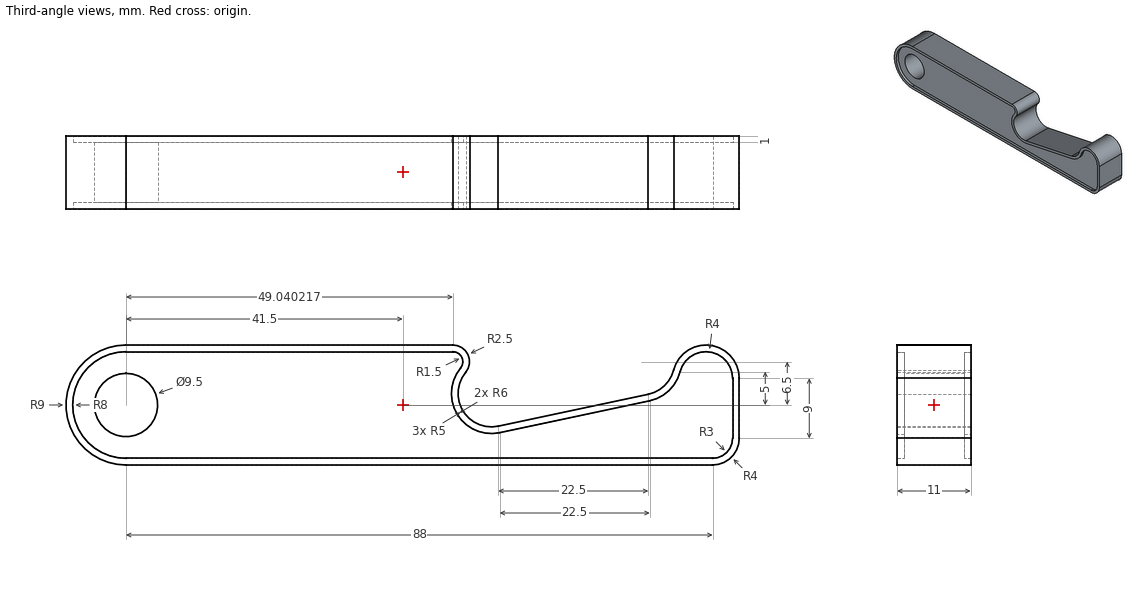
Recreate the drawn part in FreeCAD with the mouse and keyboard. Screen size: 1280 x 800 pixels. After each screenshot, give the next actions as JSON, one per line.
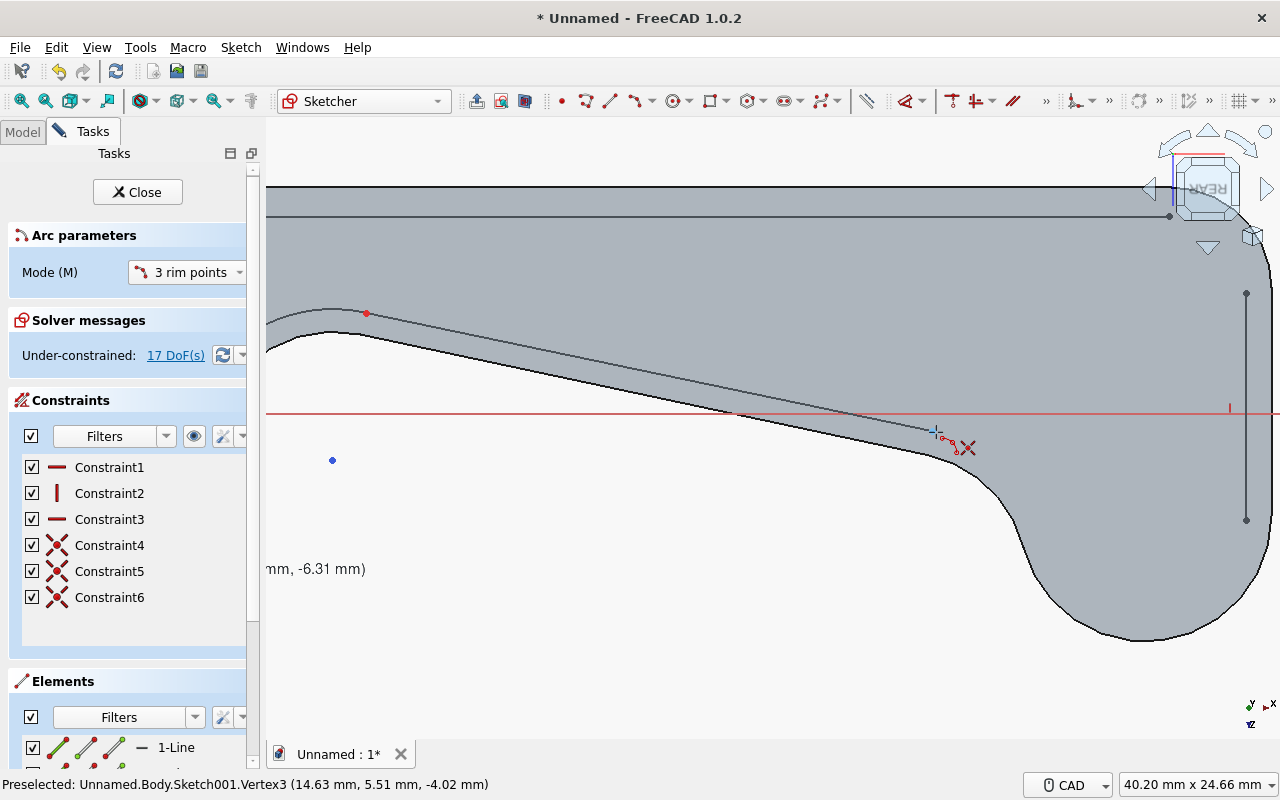
{"action": "left_click", "coordinate": [933, 431]}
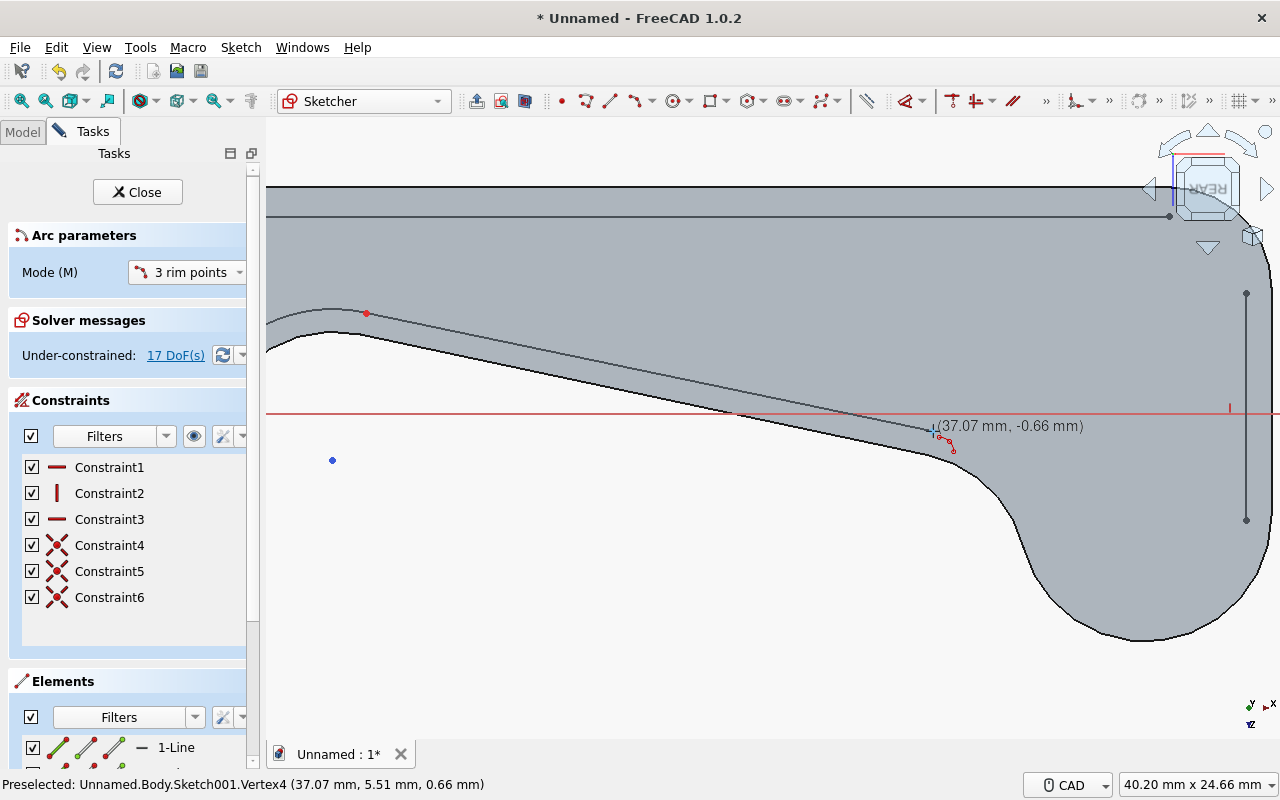
{"action": "scroll", "coordinate": [936, 432], "scroll_direction": "down", "scroll_amount": 7}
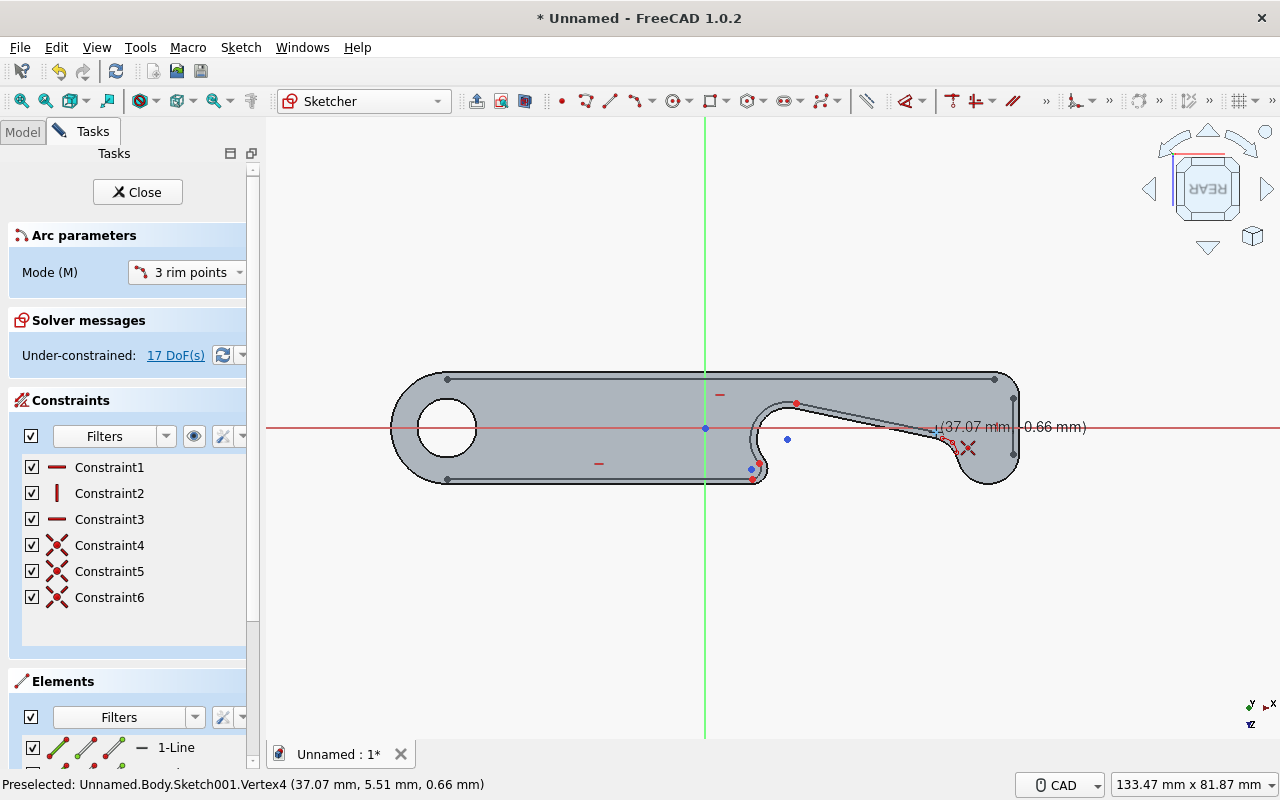
{"action": "left_click", "coordinate": [964, 459]}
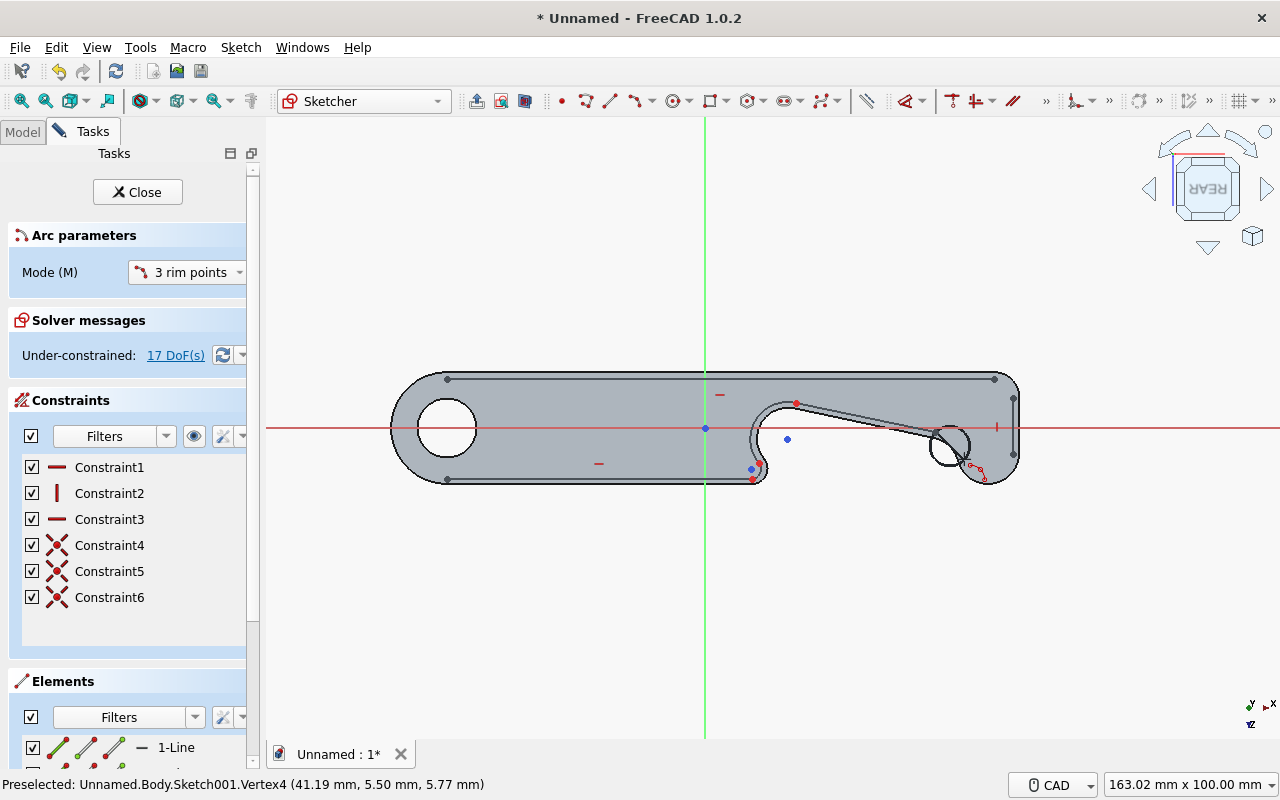
{"action": "scroll", "coordinate": [954, 442], "scroll_direction": "up", "scroll_amount": 6}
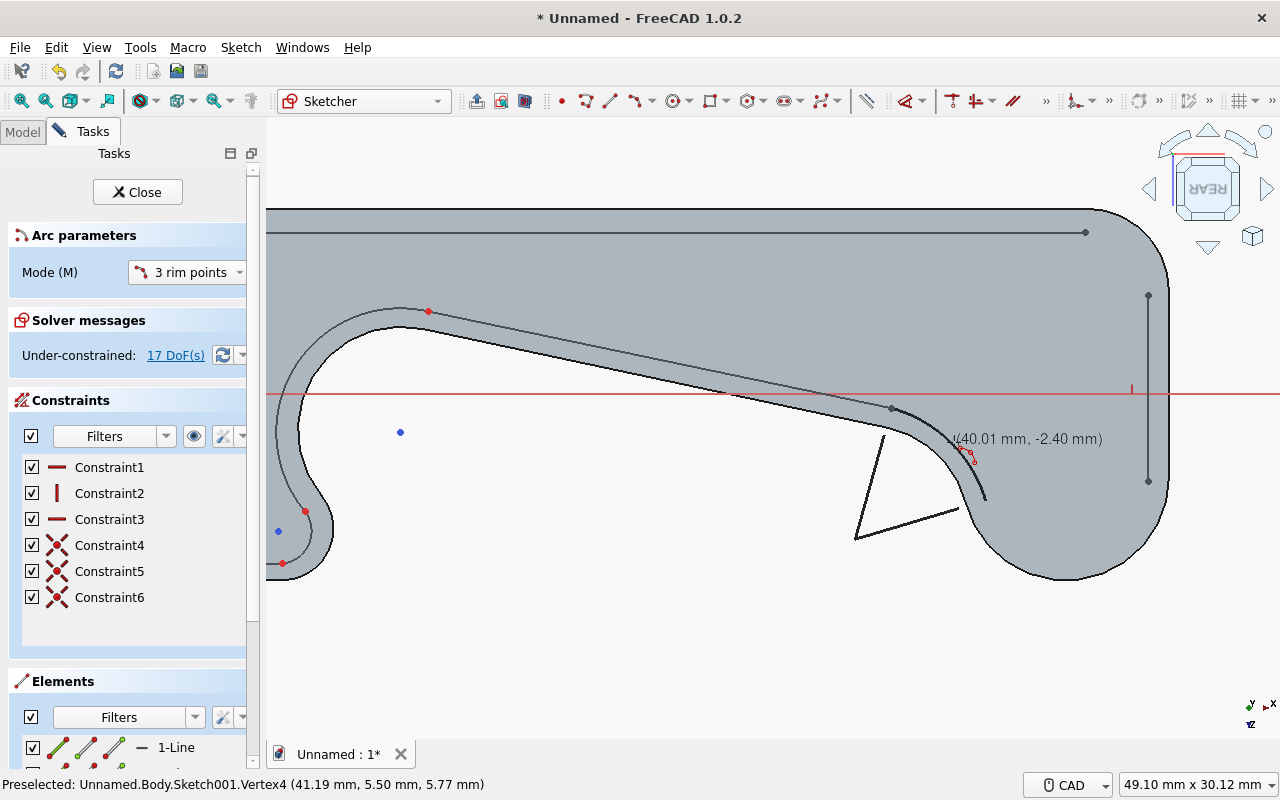
{"action": "left_click", "coordinate": [952, 439]}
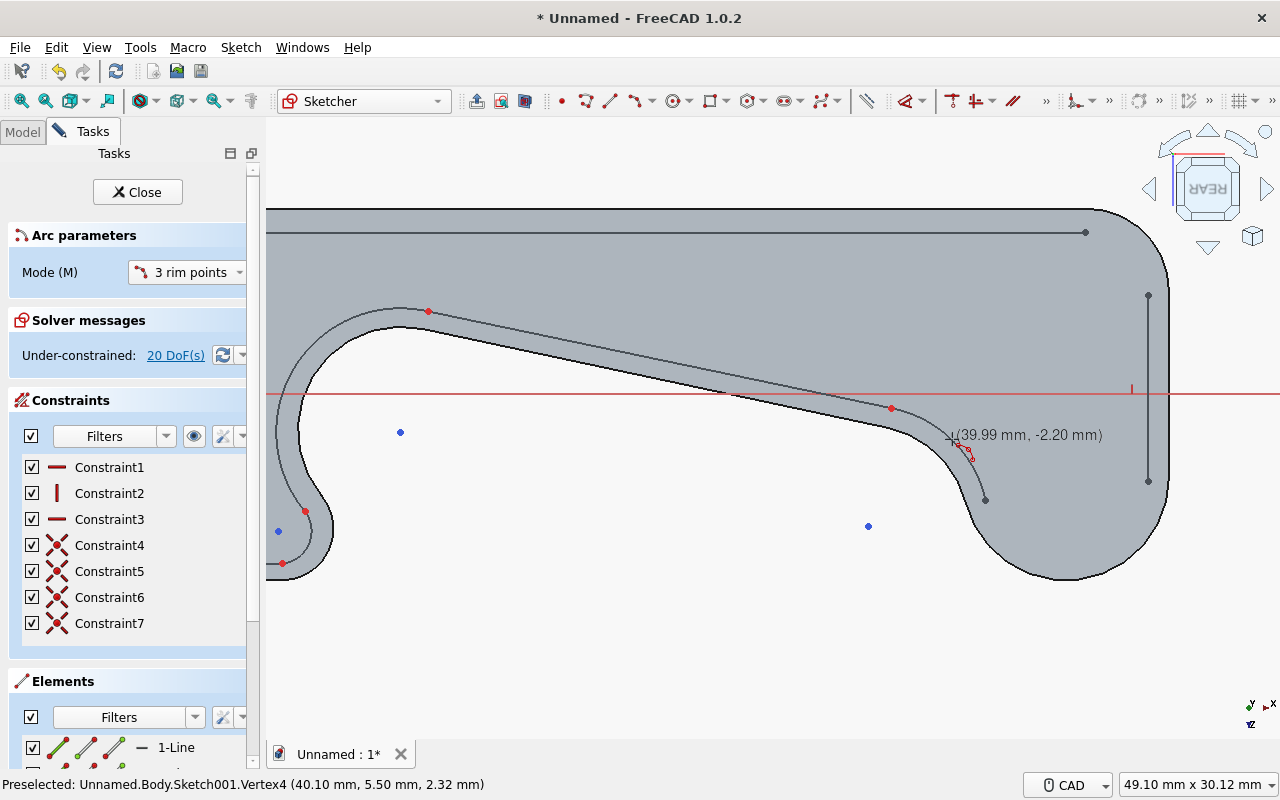
{"action": "left_click", "coordinate": [986, 501]}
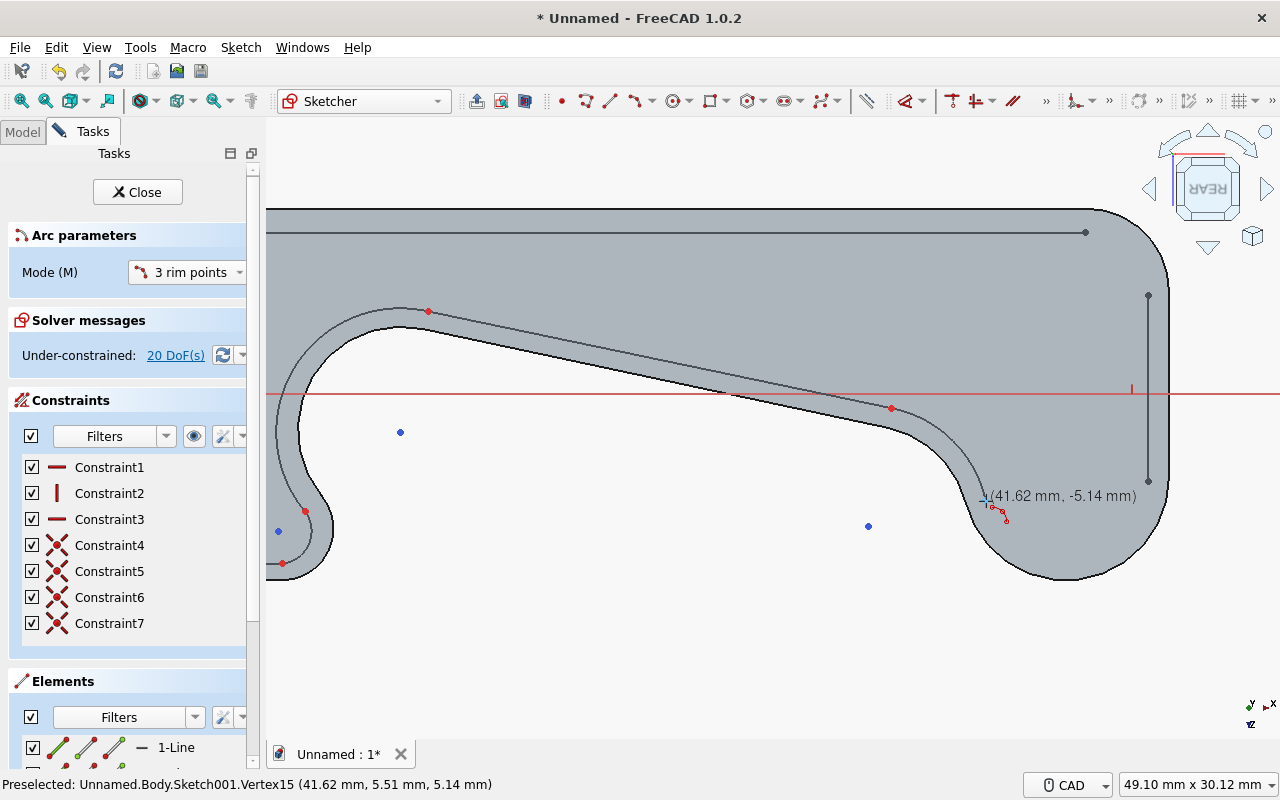
{"action": "scroll", "coordinate": [954, 442], "scroll_direction": "down", "scroll_amount": 6}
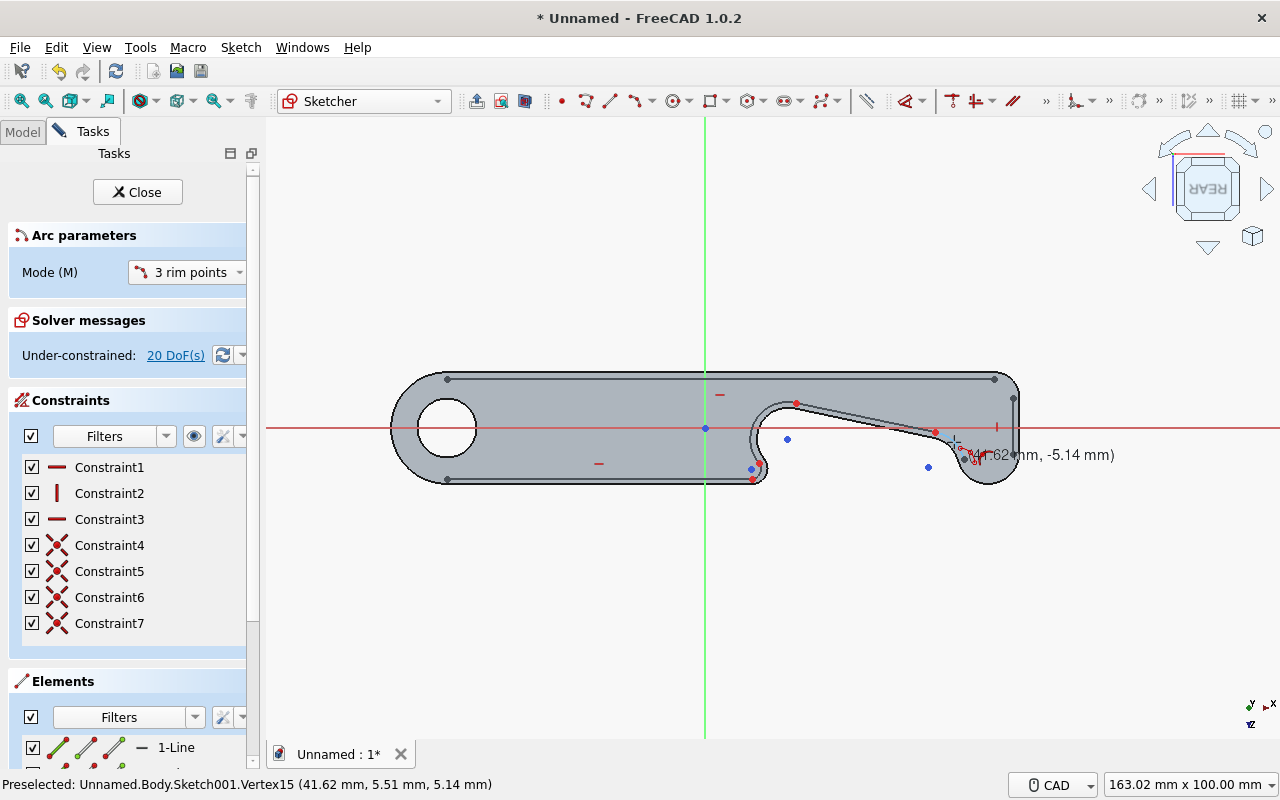
{"action": "left_click", "coordinate": [1013, 454]}
{"action": "left_click", "coordinate": [991, 478]}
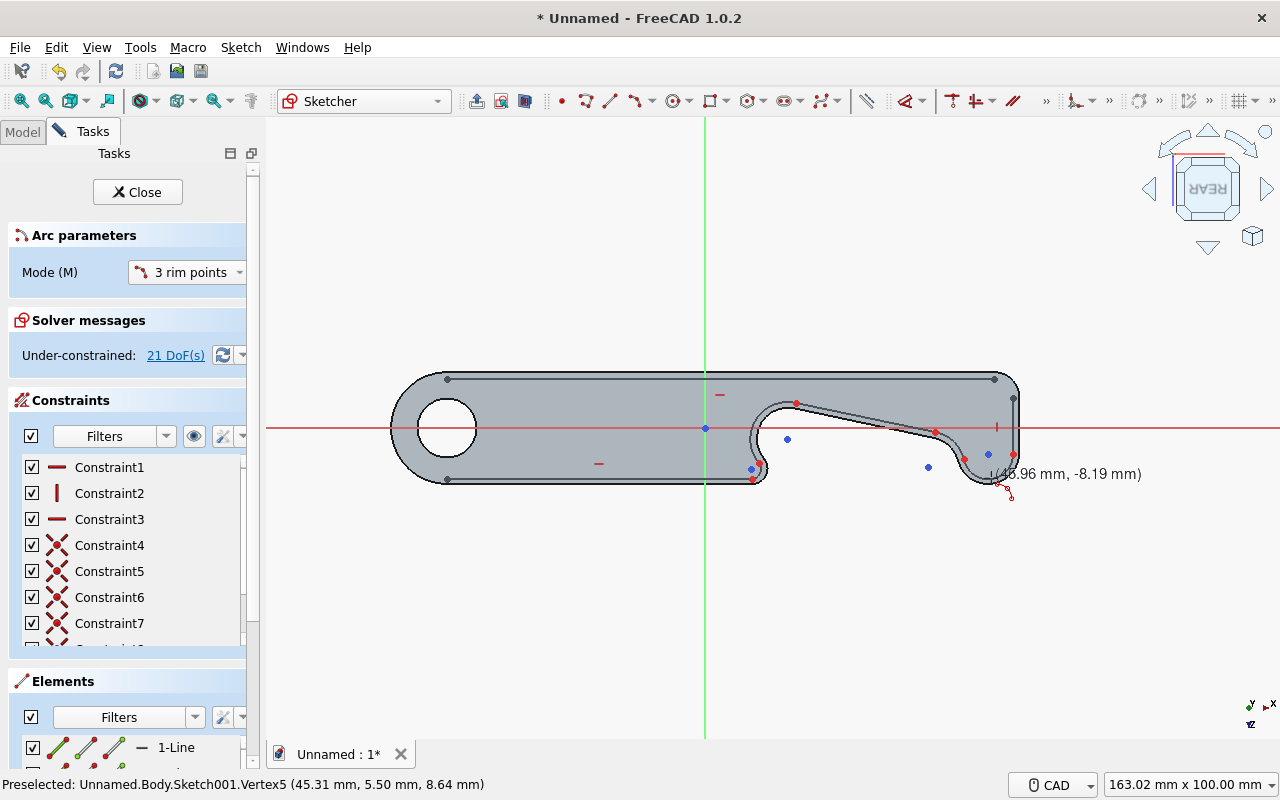
{"action": "left_click", "coordinate": [1013, 398]}
{"action": "left_click", "coordinate": [994, 379]}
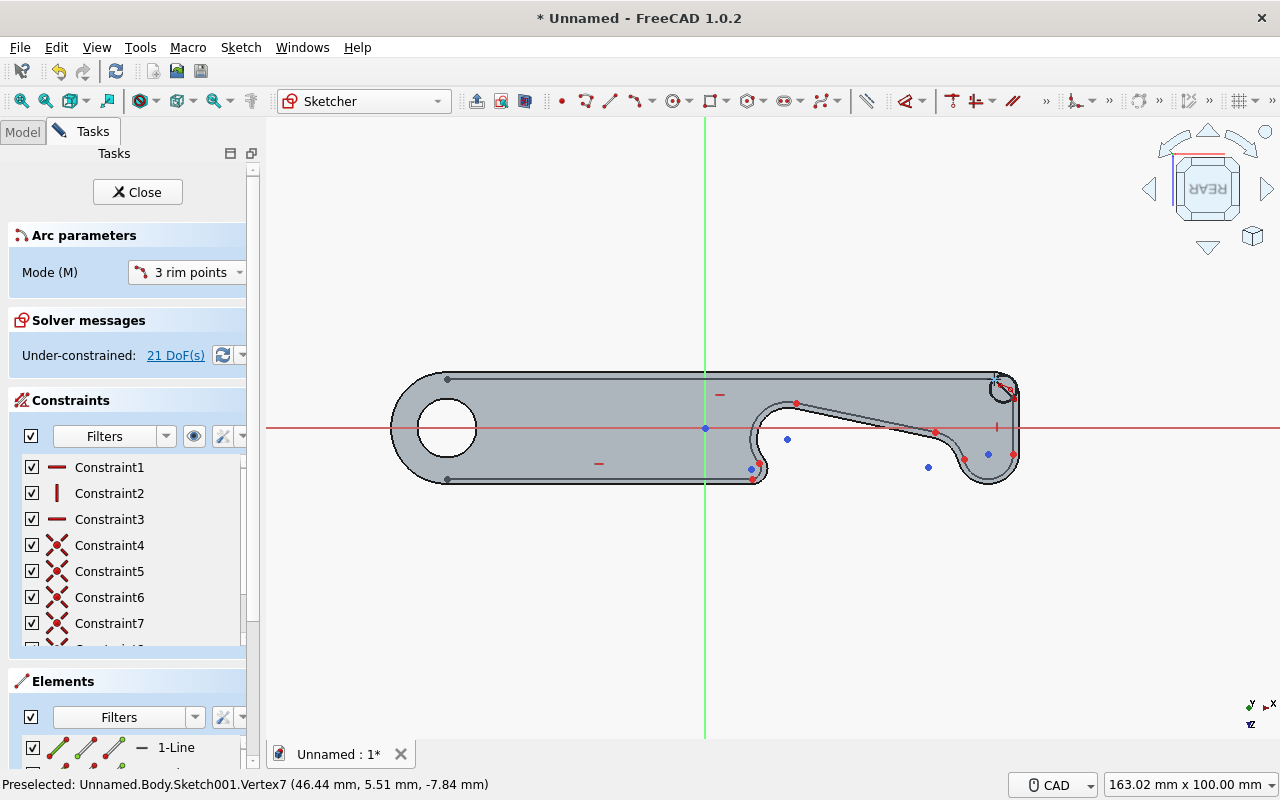
{"action": "scroll", "coordinate": [1008, 384], "scroll_direction": "up", "scroll_amount": 6}